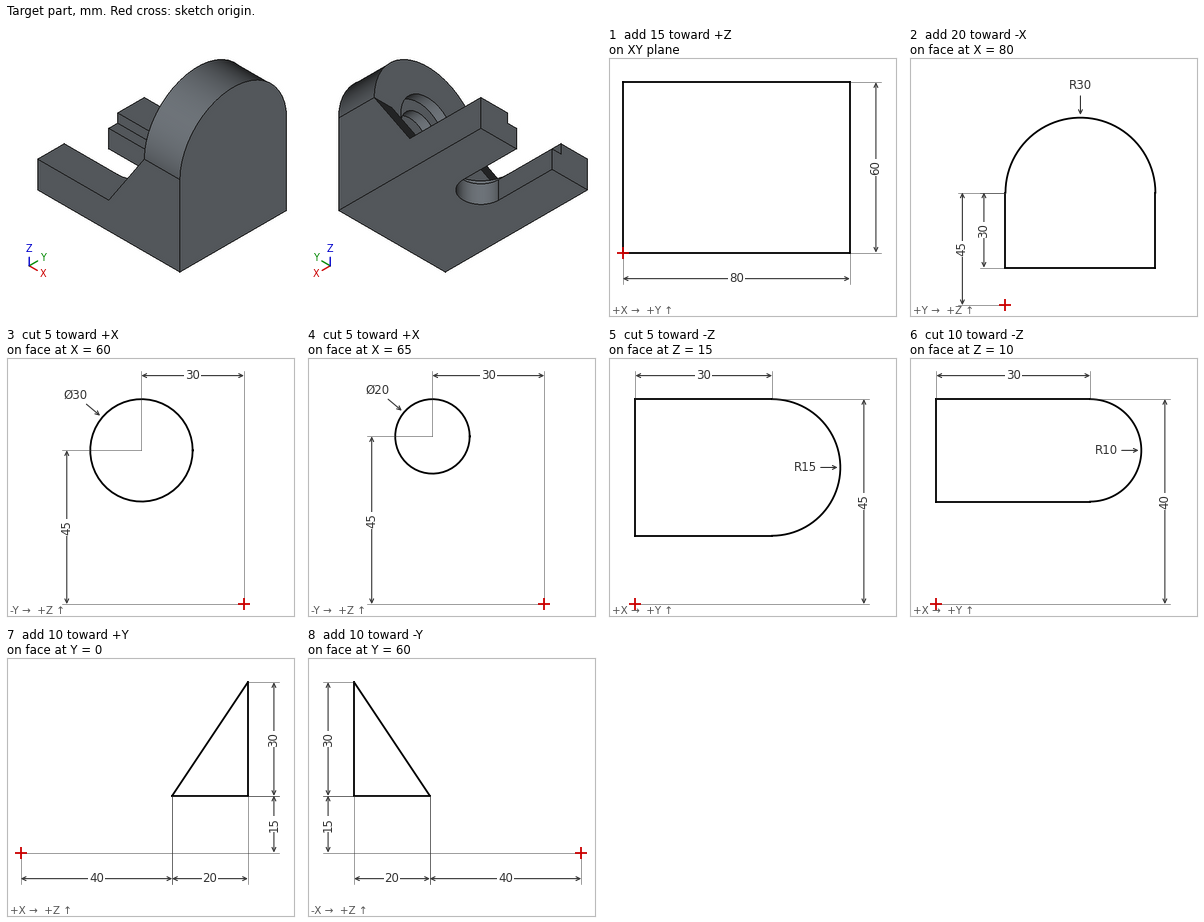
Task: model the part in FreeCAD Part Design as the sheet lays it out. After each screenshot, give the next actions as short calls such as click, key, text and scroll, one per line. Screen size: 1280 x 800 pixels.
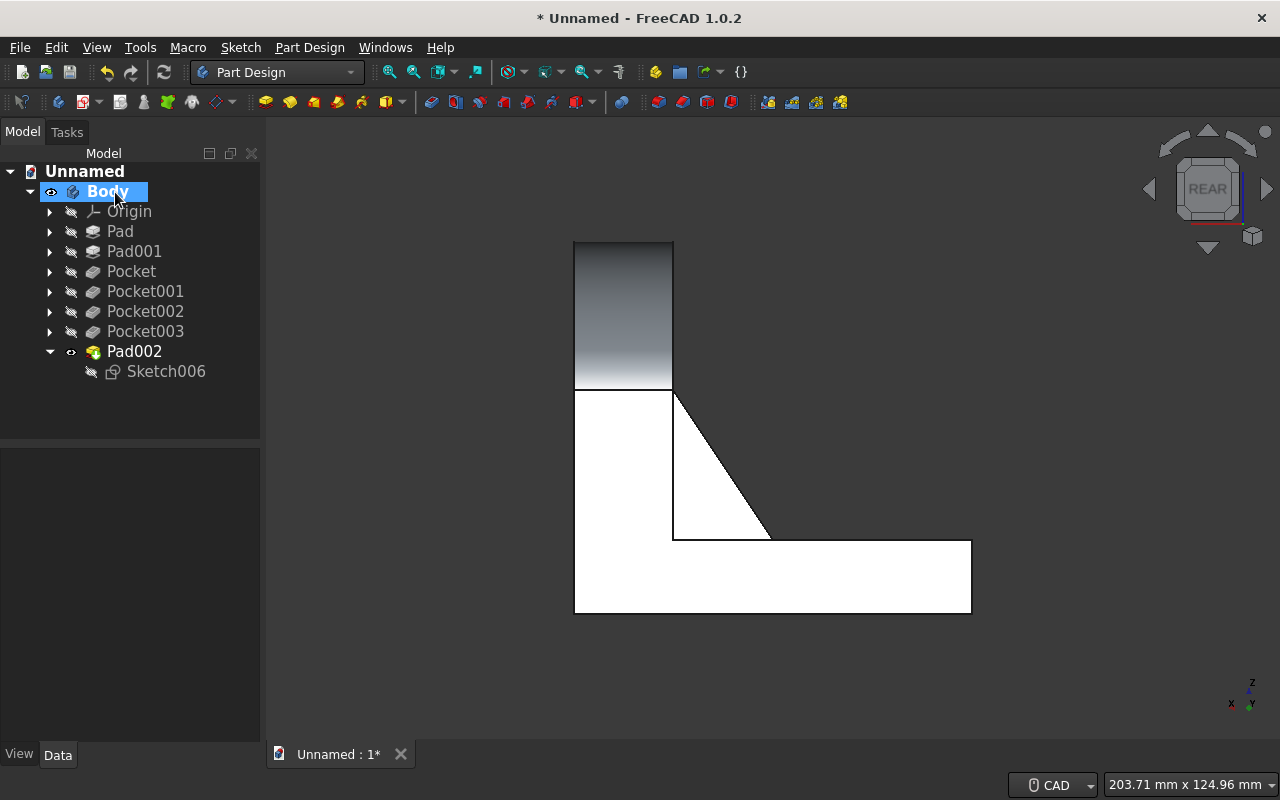
click(659, 565)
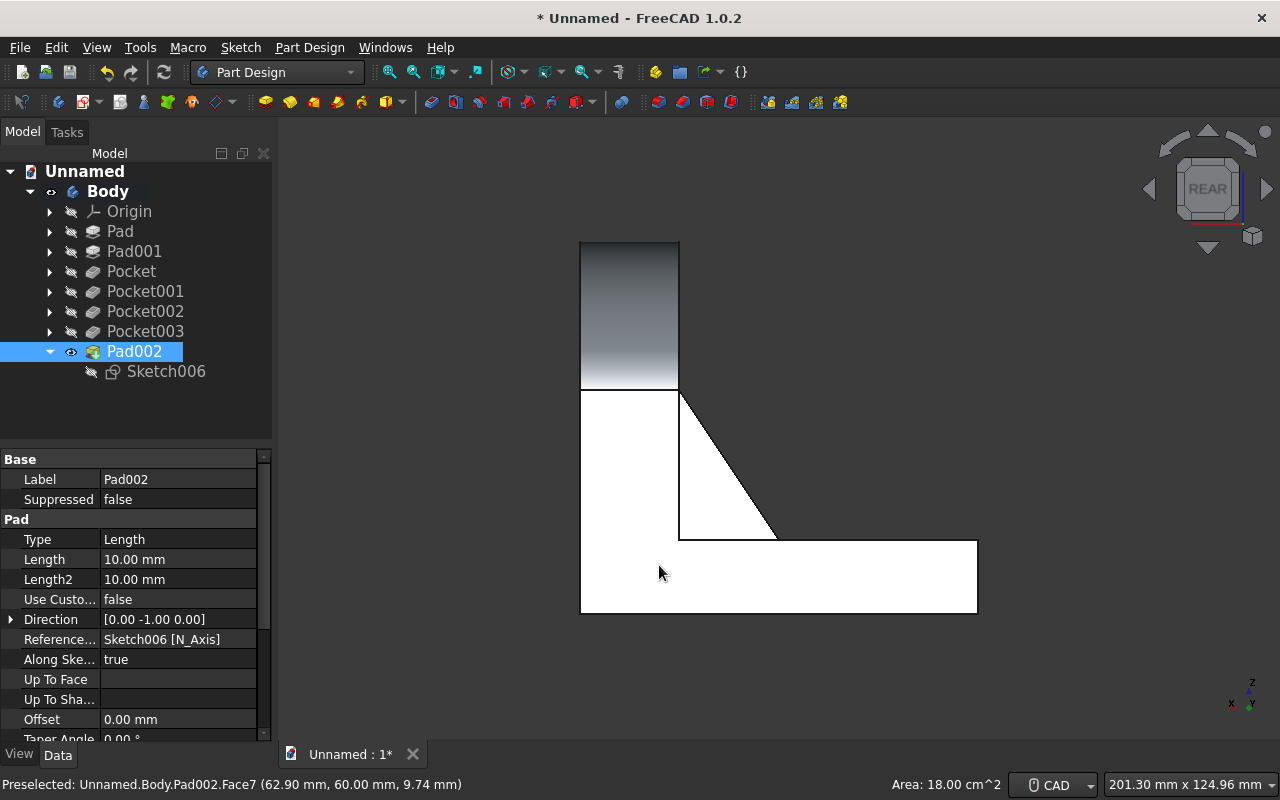
click(84, 102)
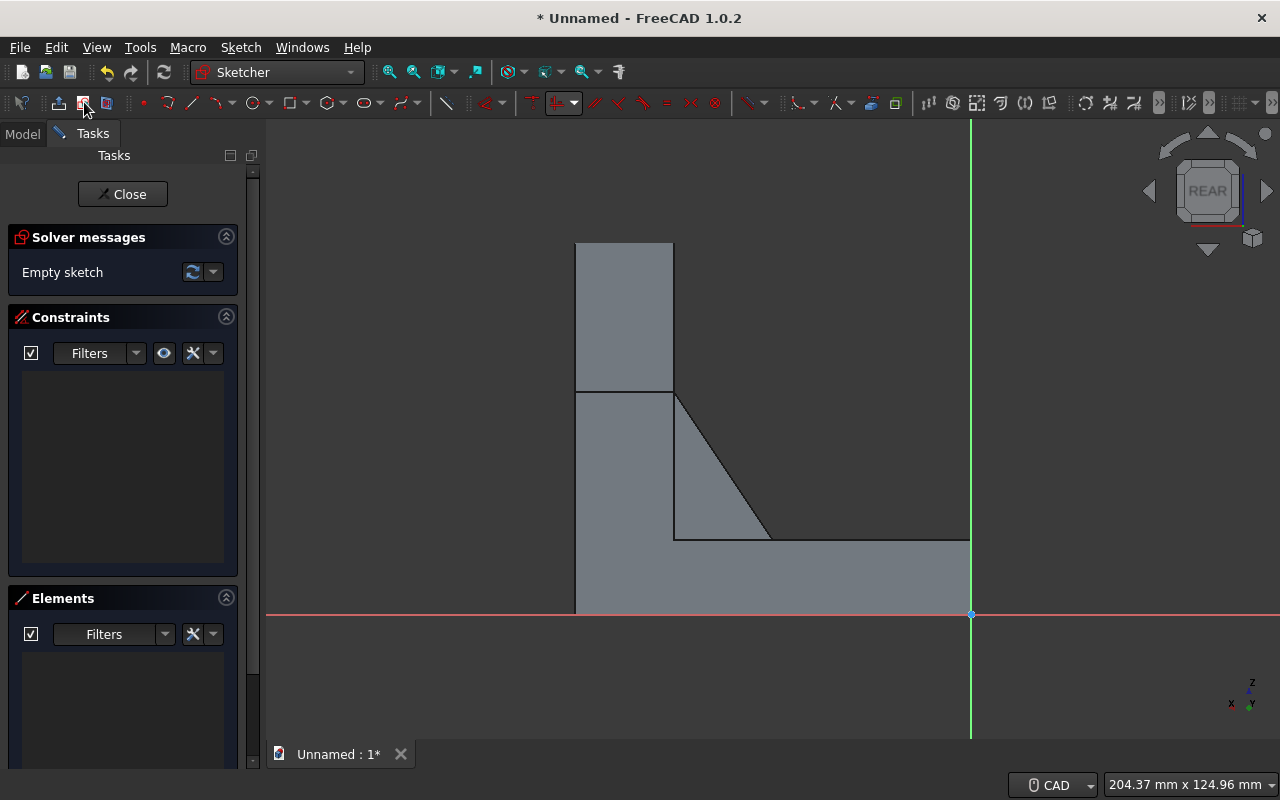
scroll(966, 594, up, 3)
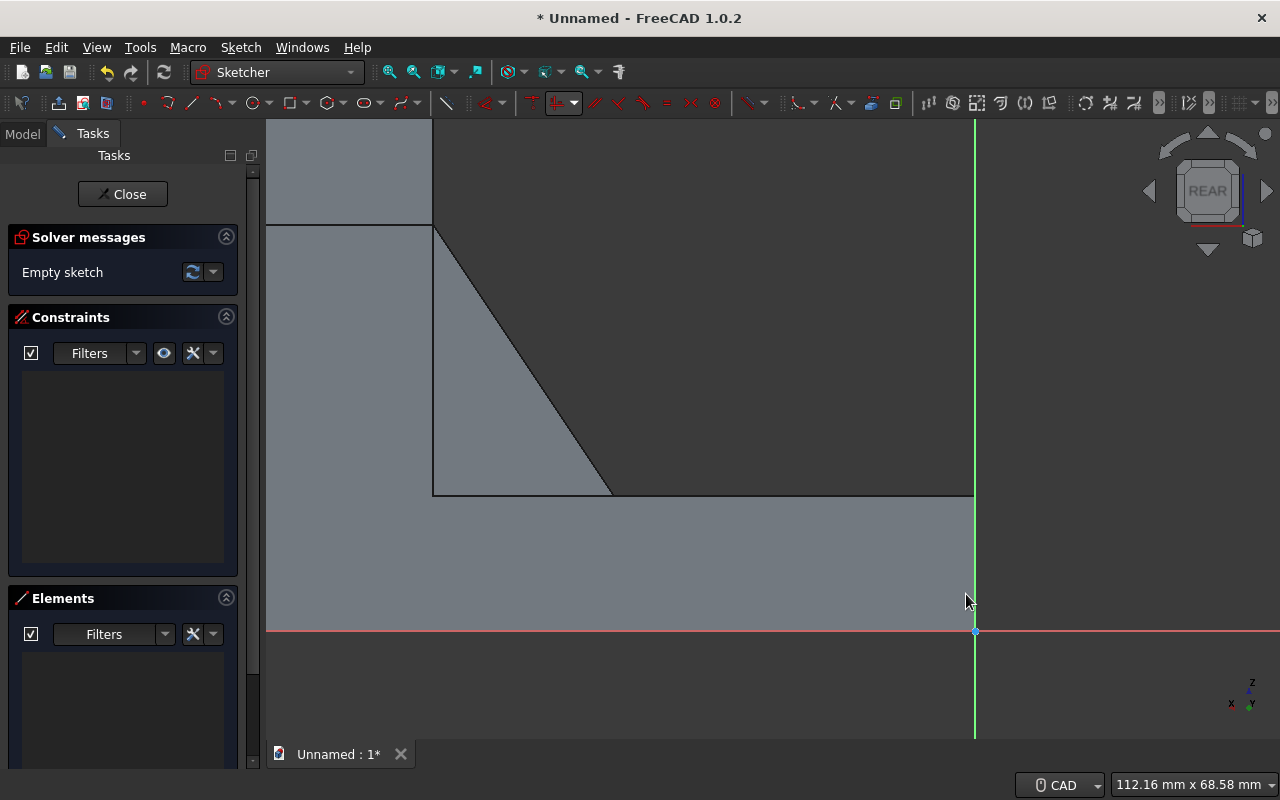
click(168, 104)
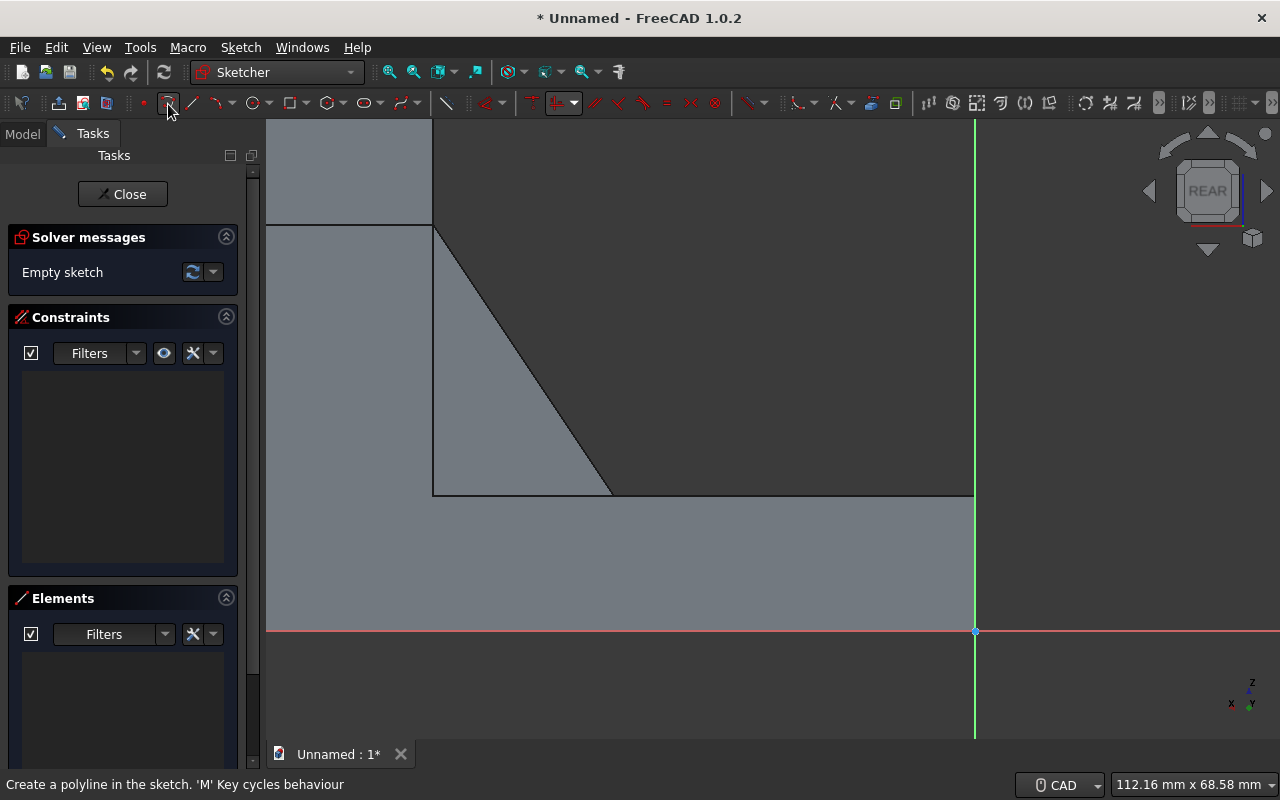
click(614, 496)
click(433, 225)
click(433, 496)
click(614, 497)
key(Escape)
key(Escape)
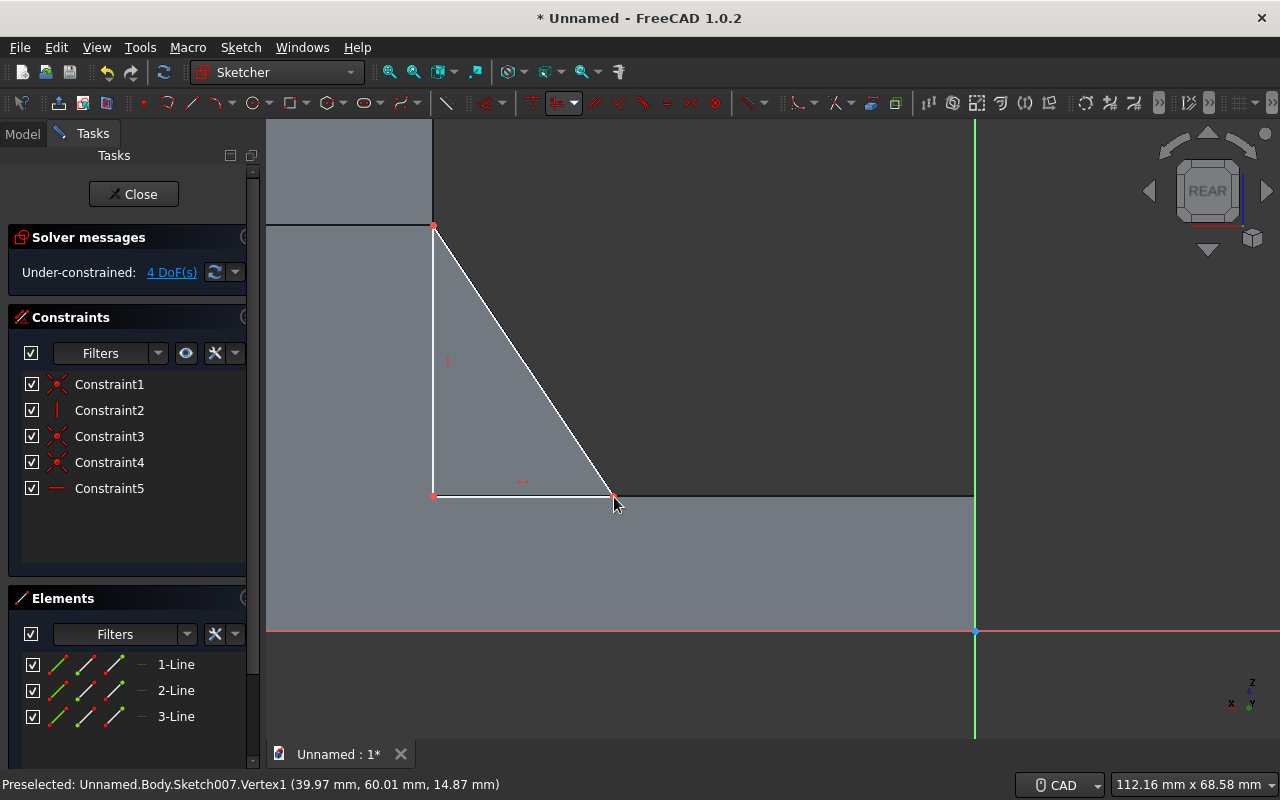
click(486, 104)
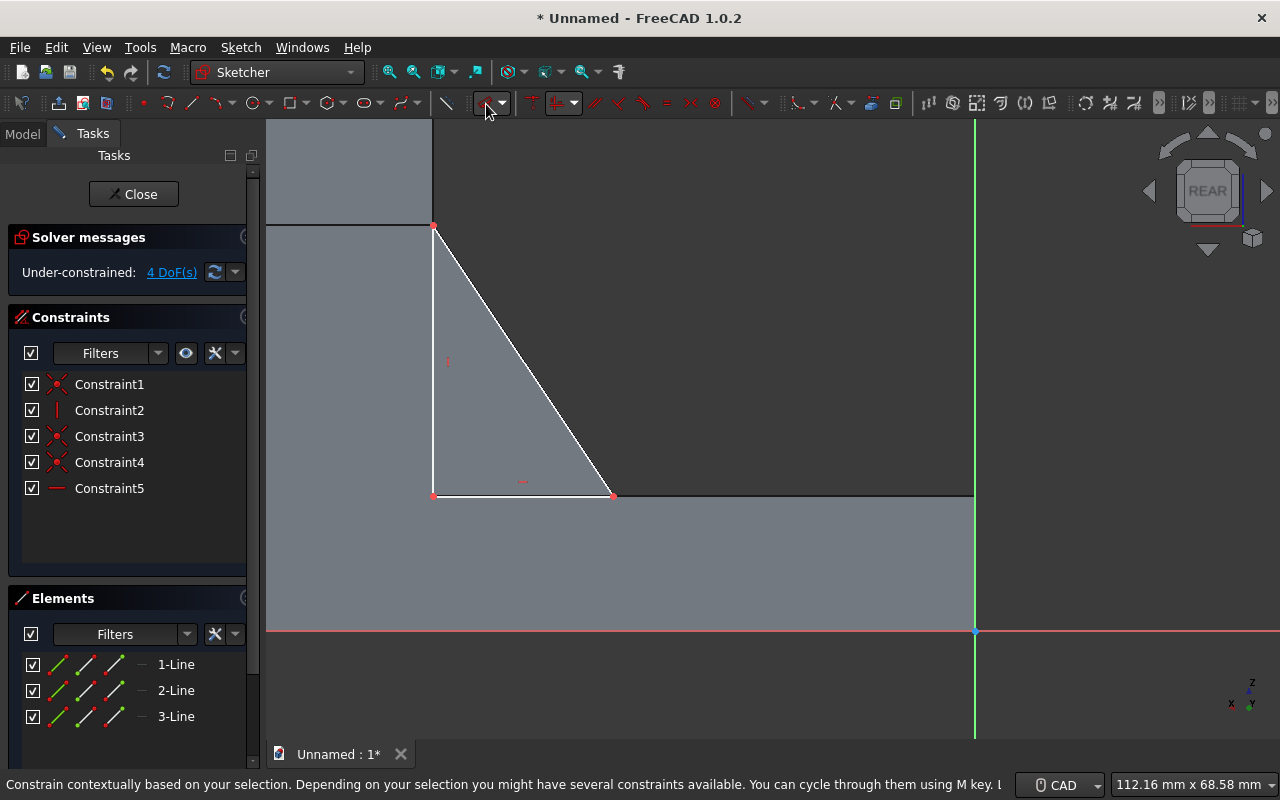
click(433, 307)
click(399, 362)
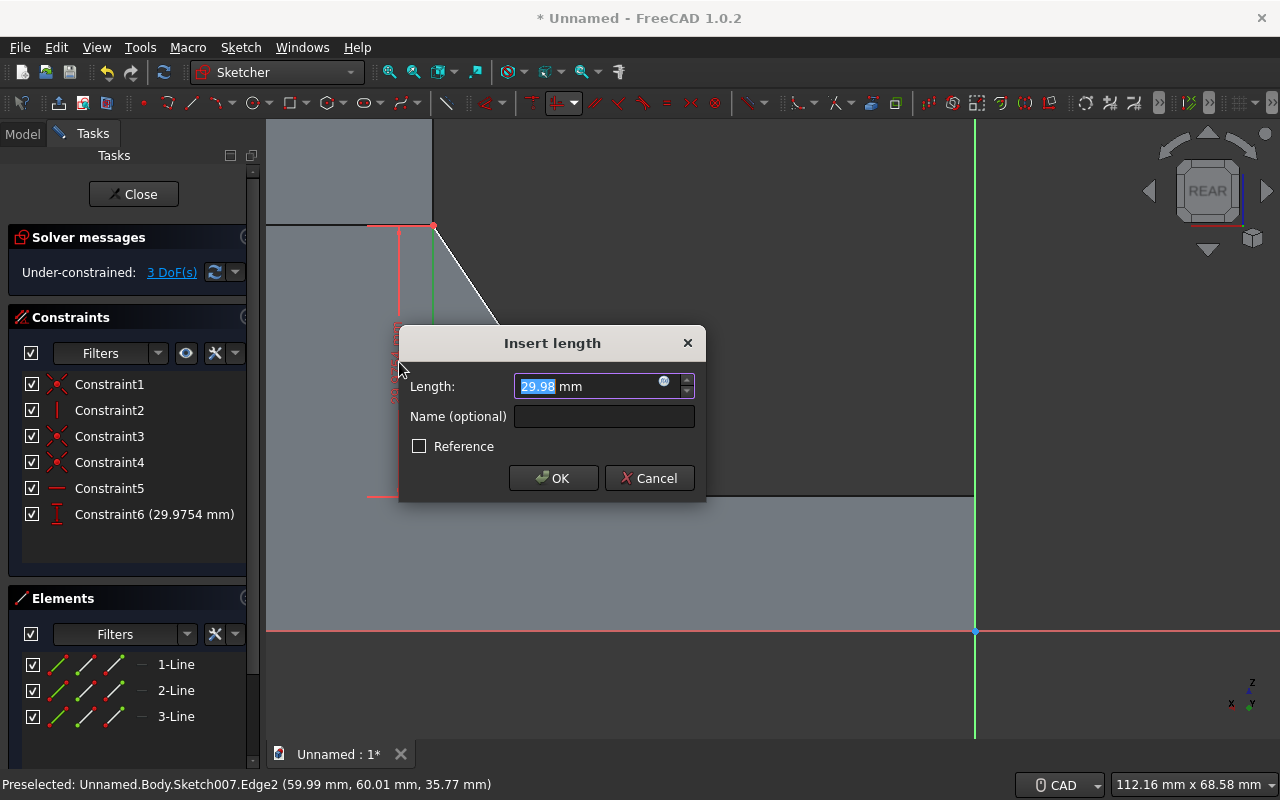
text(30)
key(Return)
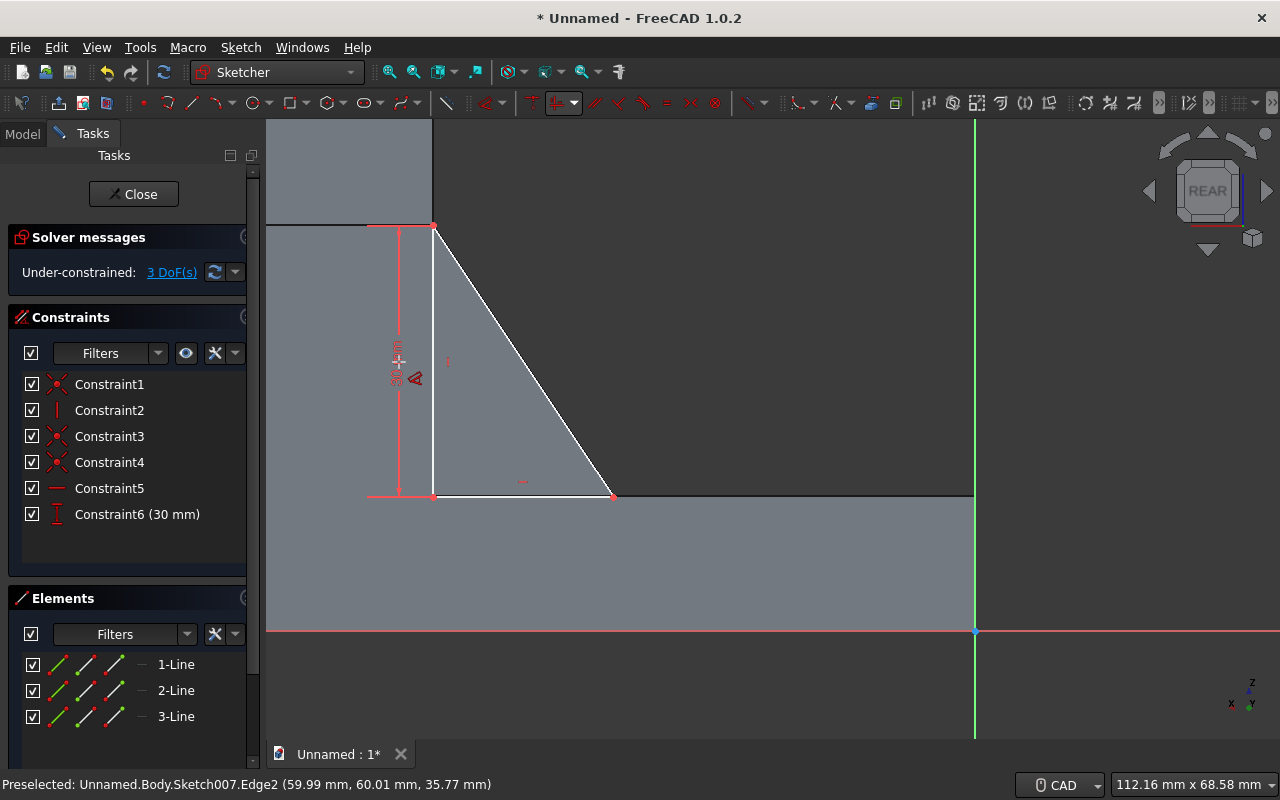
click(487, 497)
click(523, 531)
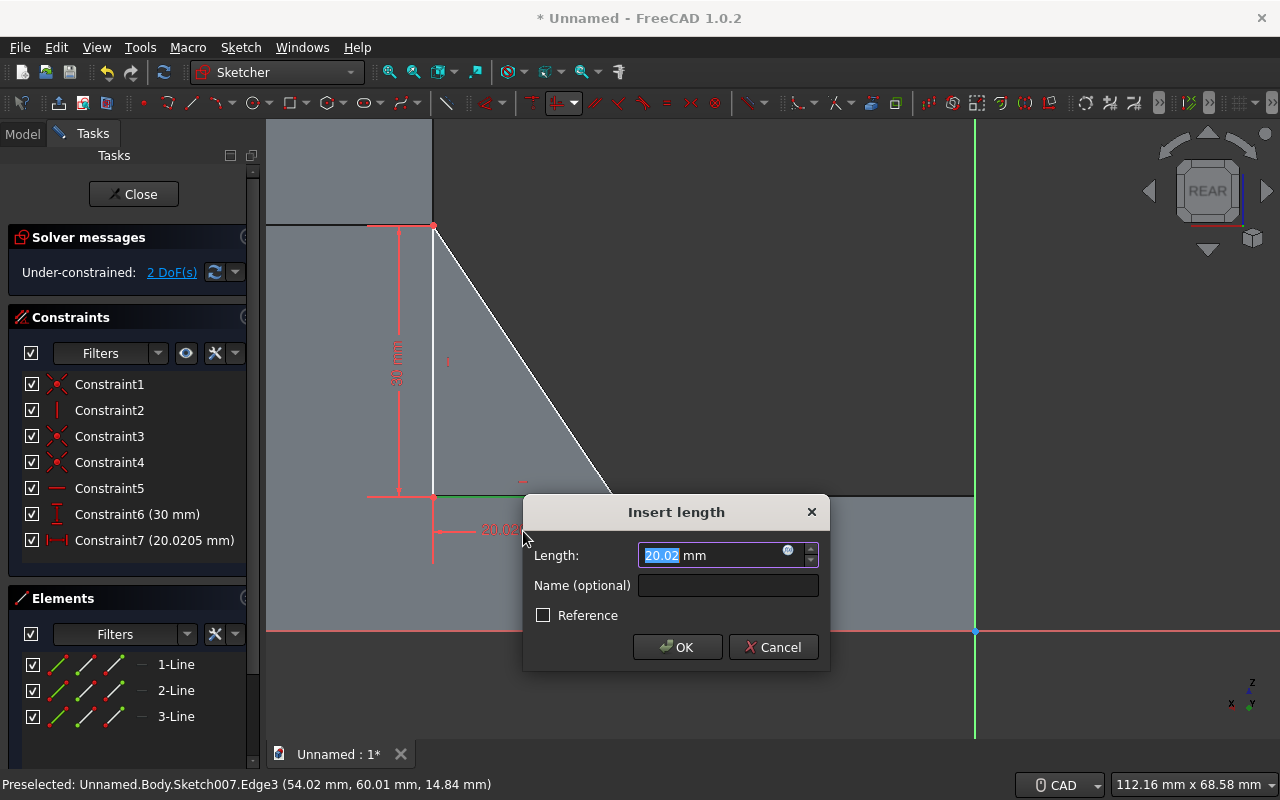
text(20)
key(Return)